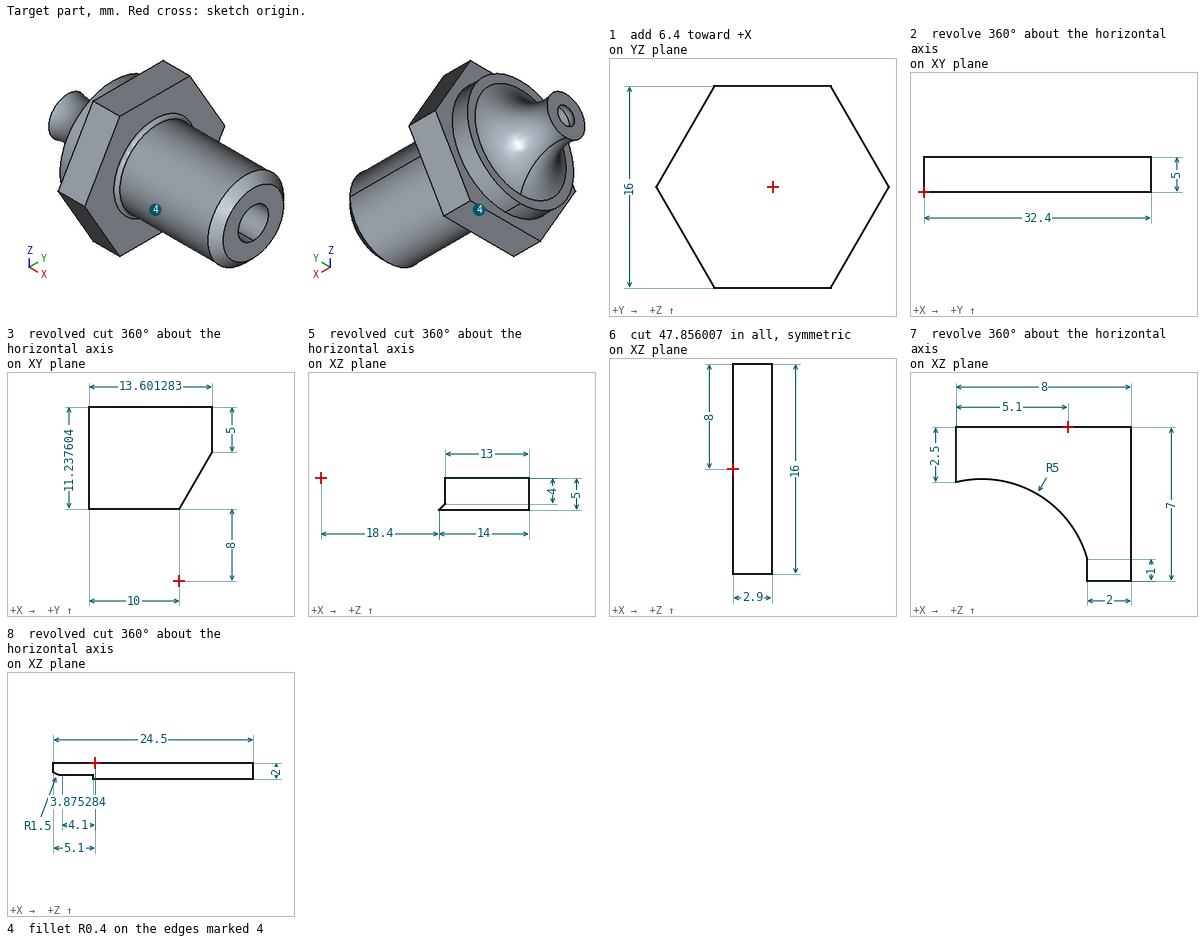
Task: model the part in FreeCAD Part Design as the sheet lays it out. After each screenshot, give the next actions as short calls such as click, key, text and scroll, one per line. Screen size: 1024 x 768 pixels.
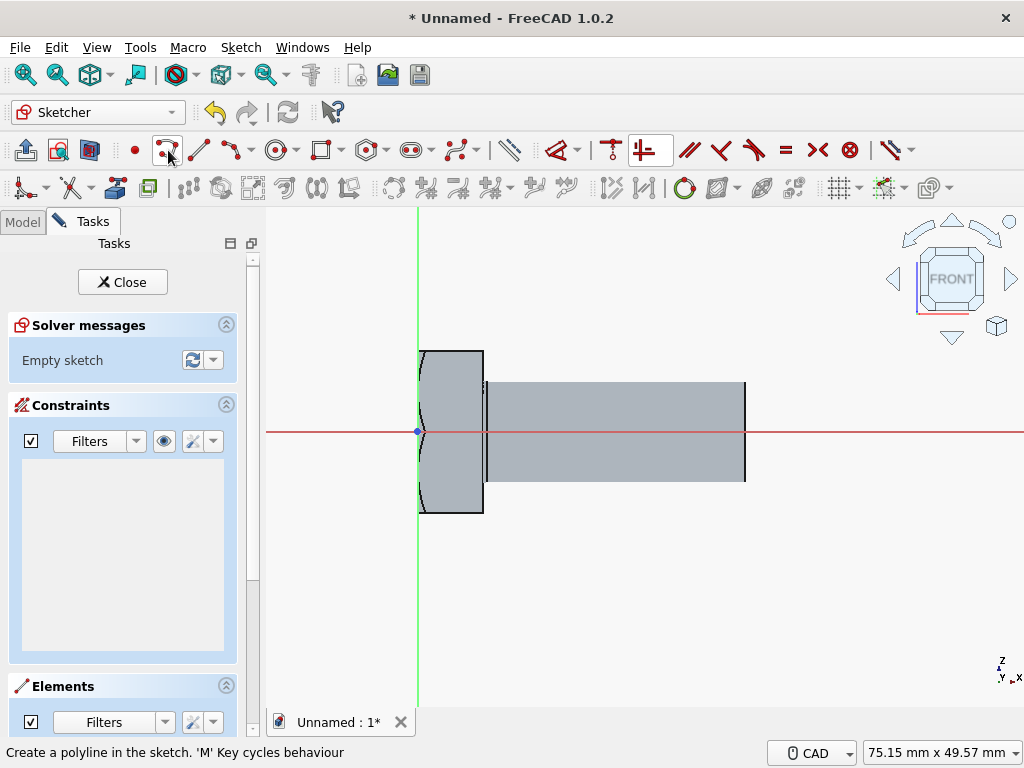
click(604, 482)
click(614, 472)
click(614, 432)
click(745, 441)
click(745, 482)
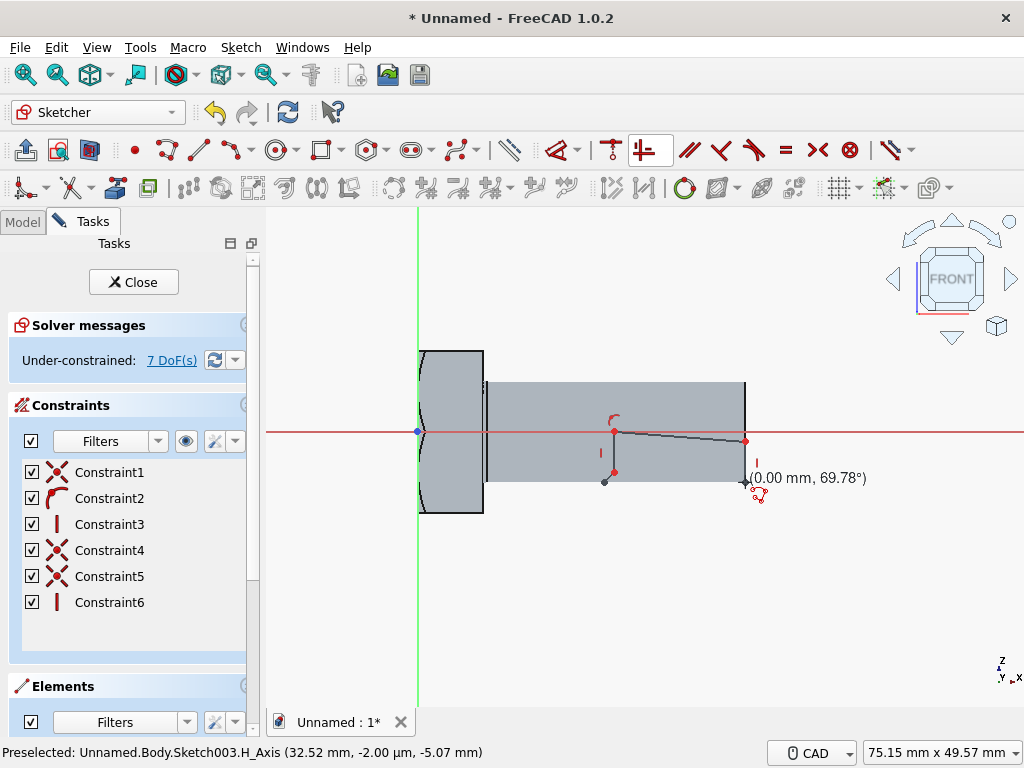
scroll(604, 482, up, 5)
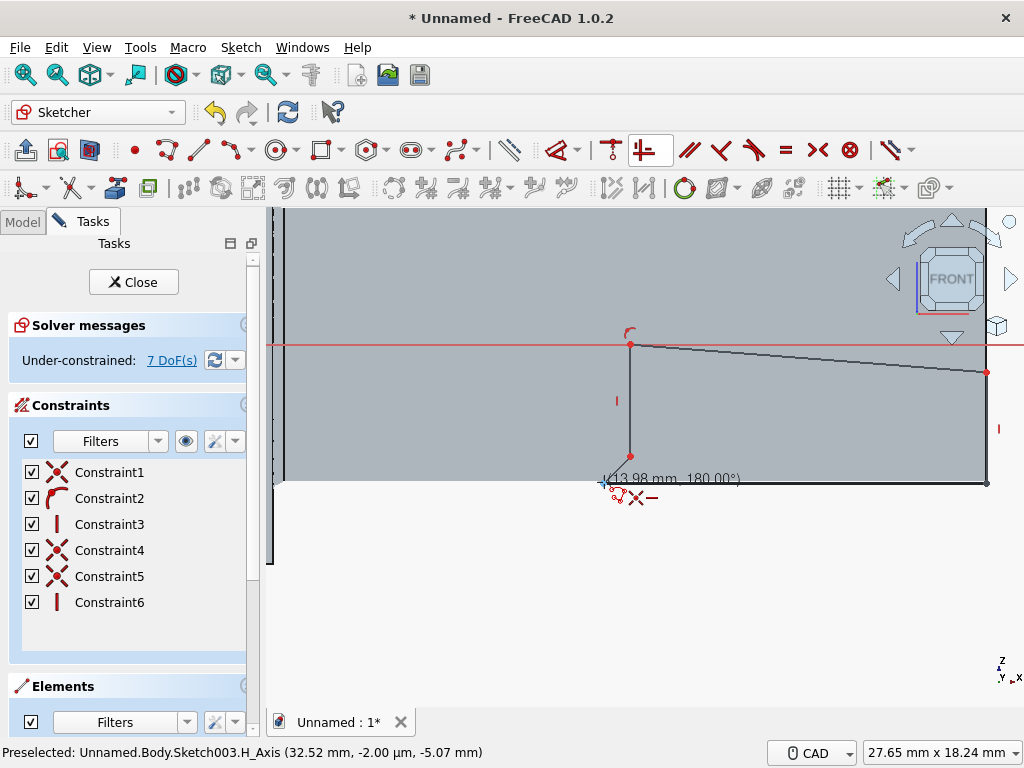
click(603, 484)
key(Escape)
key(Escape)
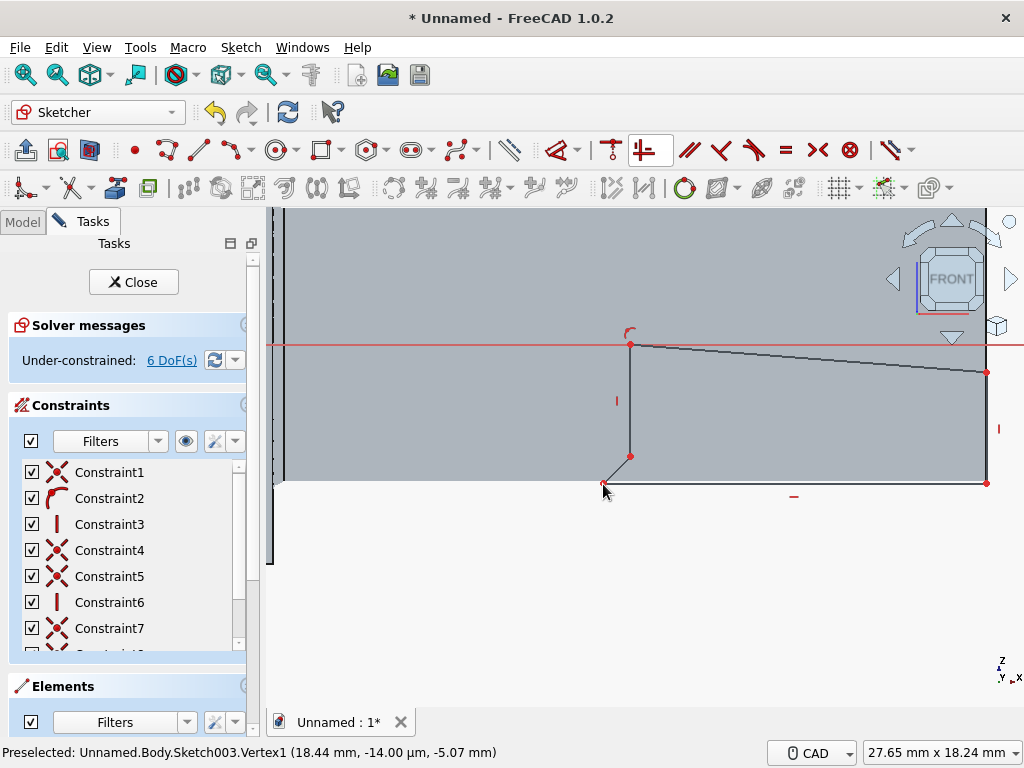
scroll(773, 356, up, 2)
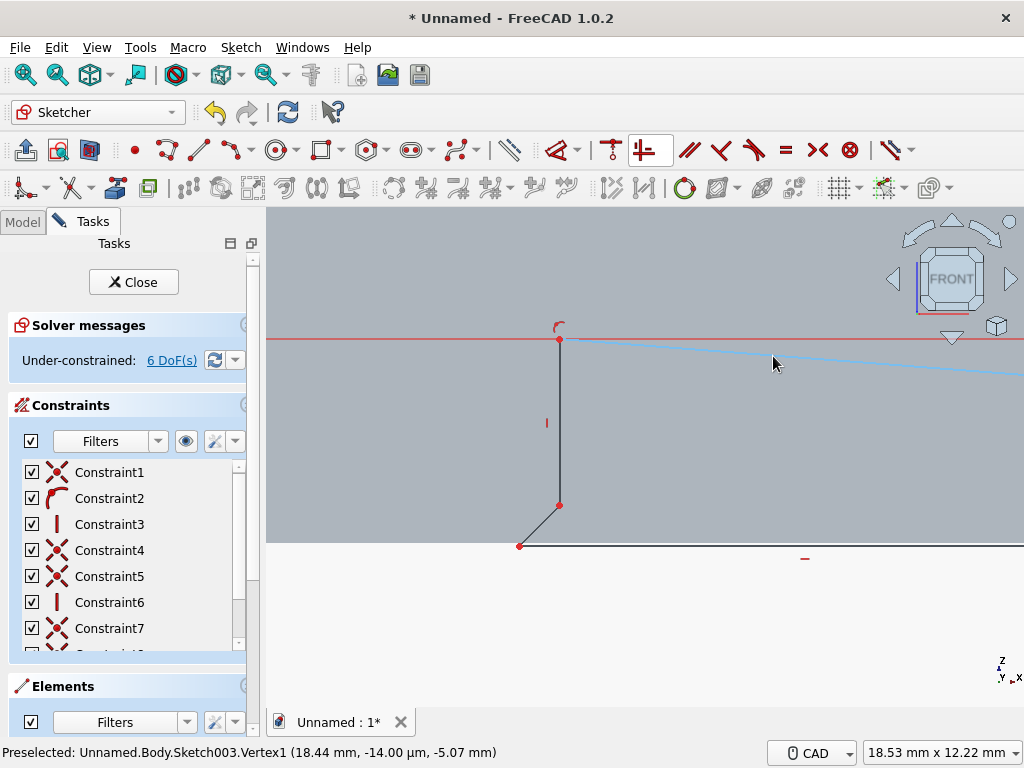
click(772, 355)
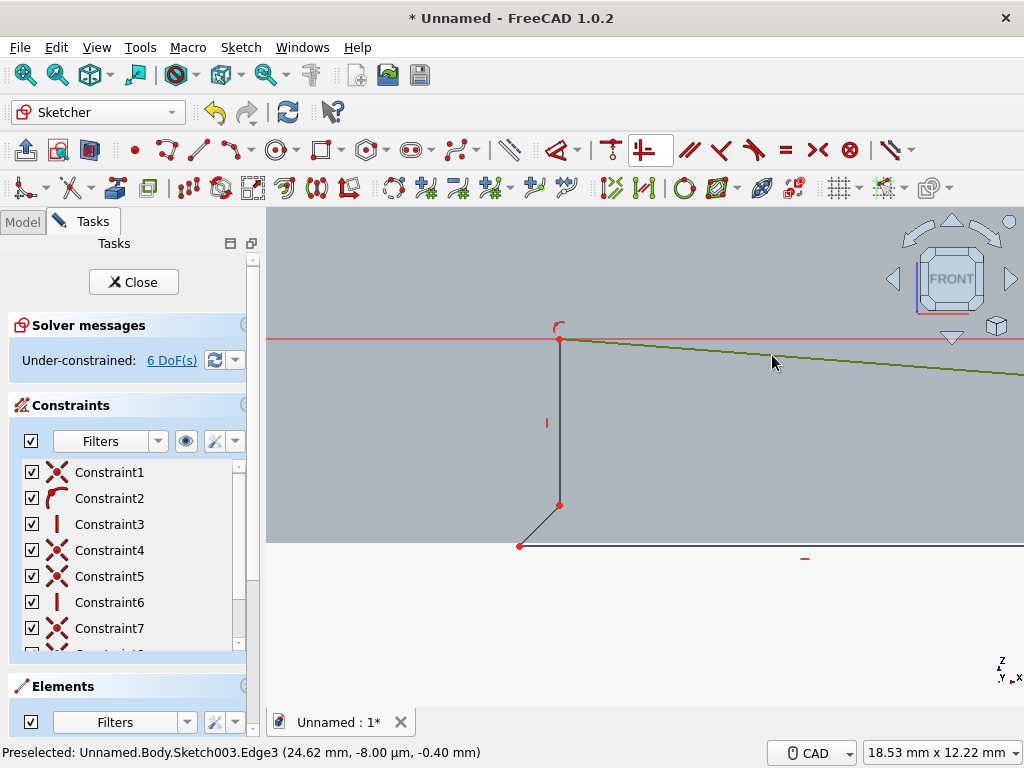
key(h)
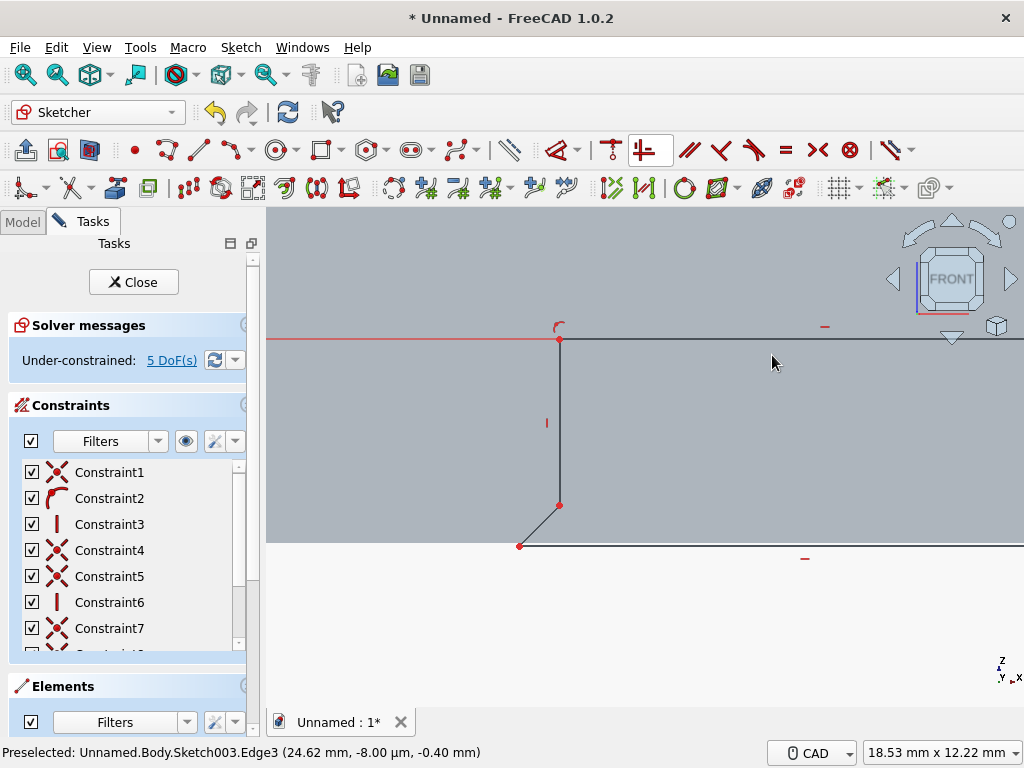
click(556, 150)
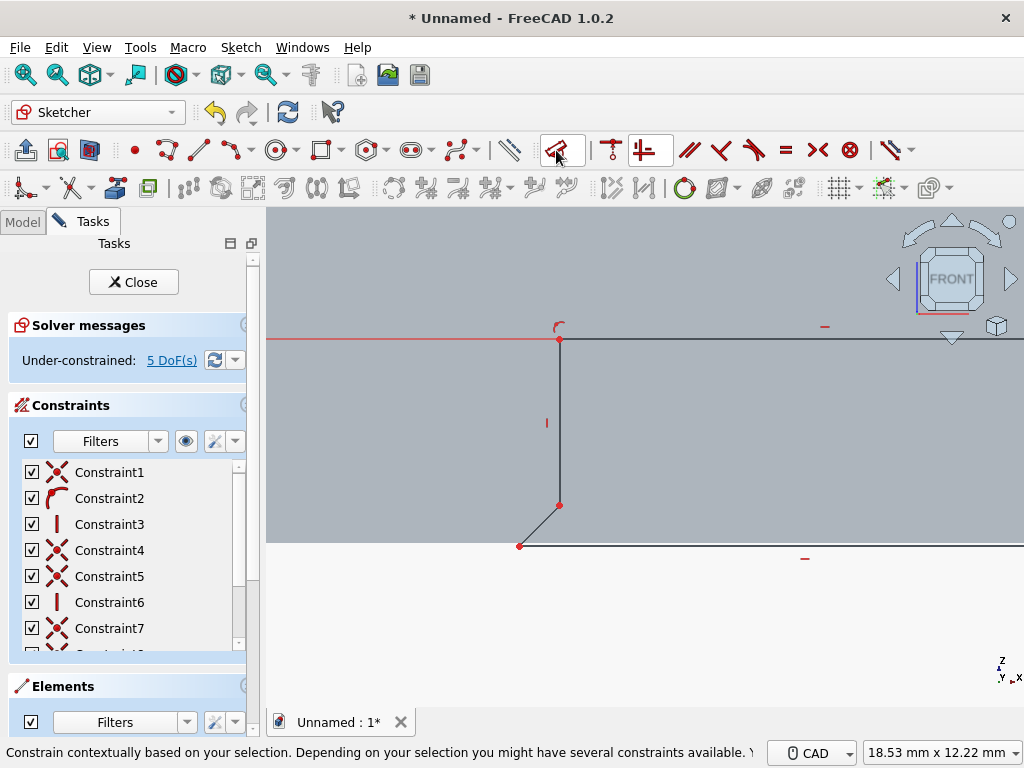
scroll(641, 464, down, 6)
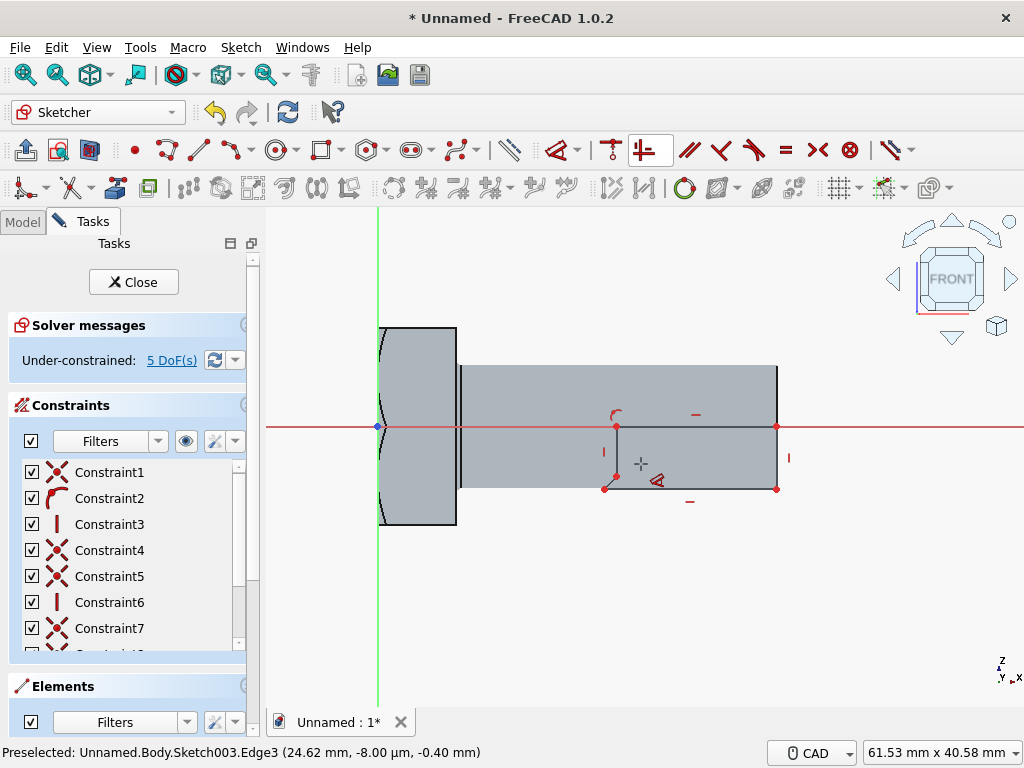
click(617, 462)
click(651, 452)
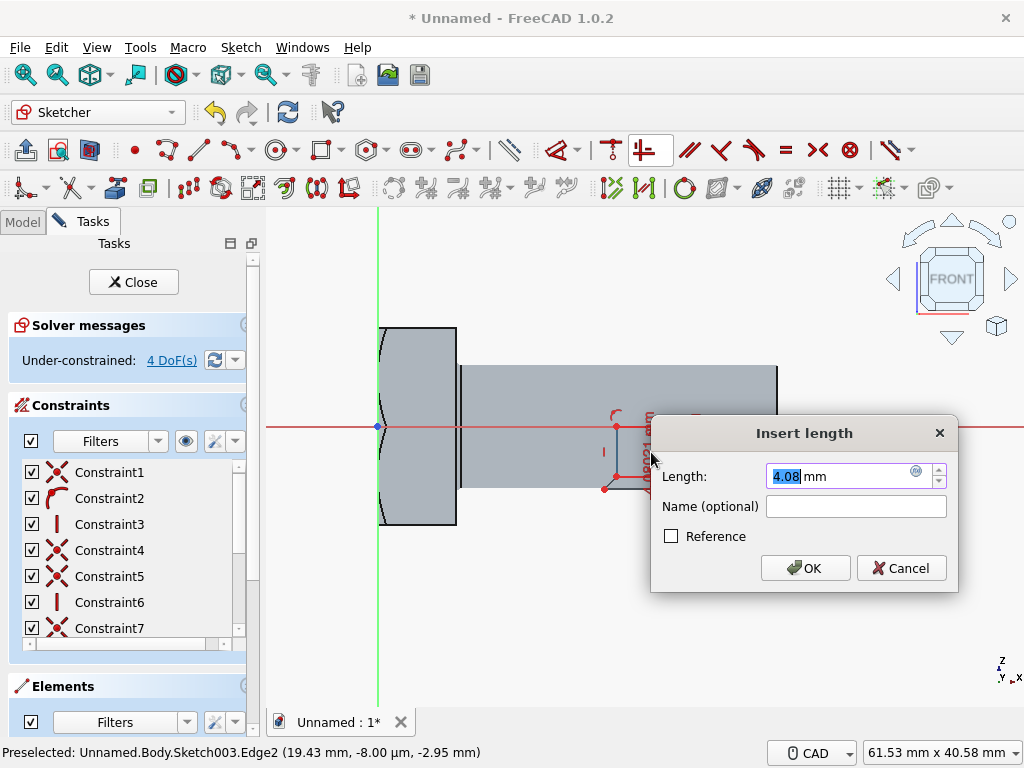
text(4)
key(Return)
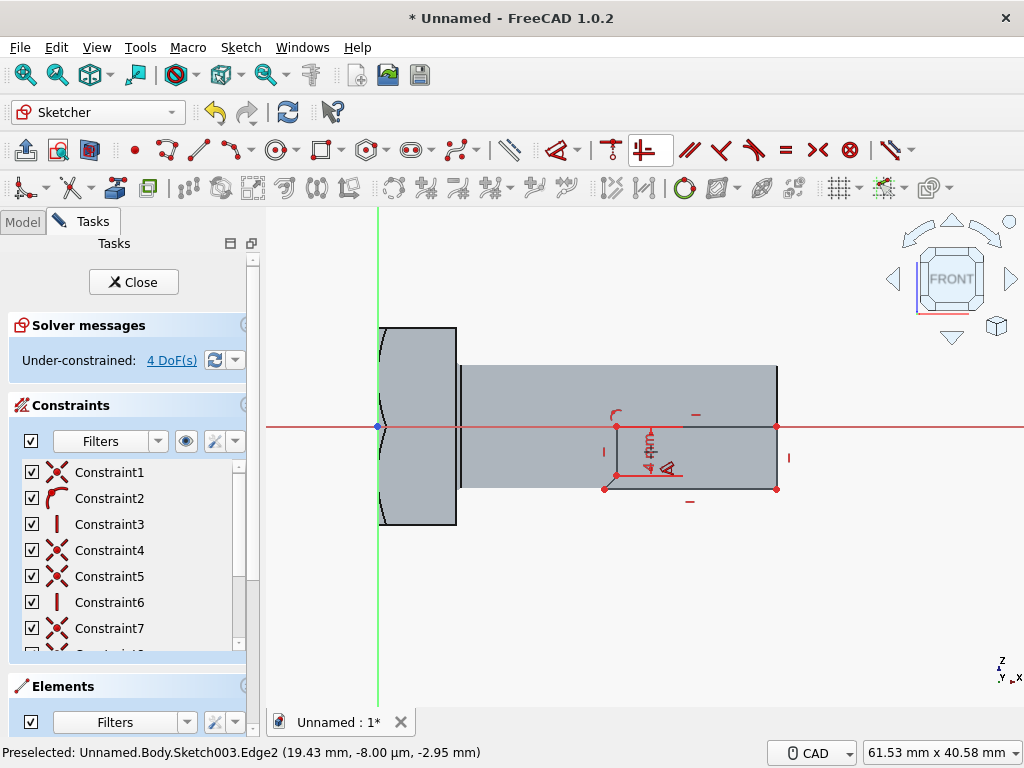
click(777, 445)
click(811, 458)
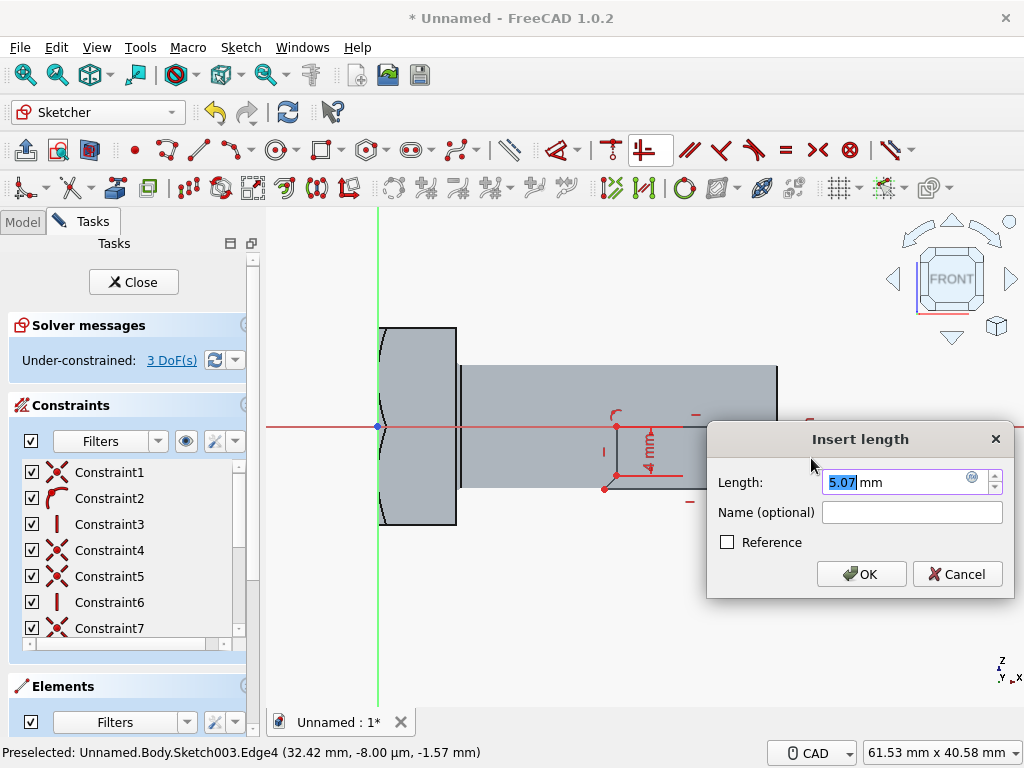
text(5)
key(Return)